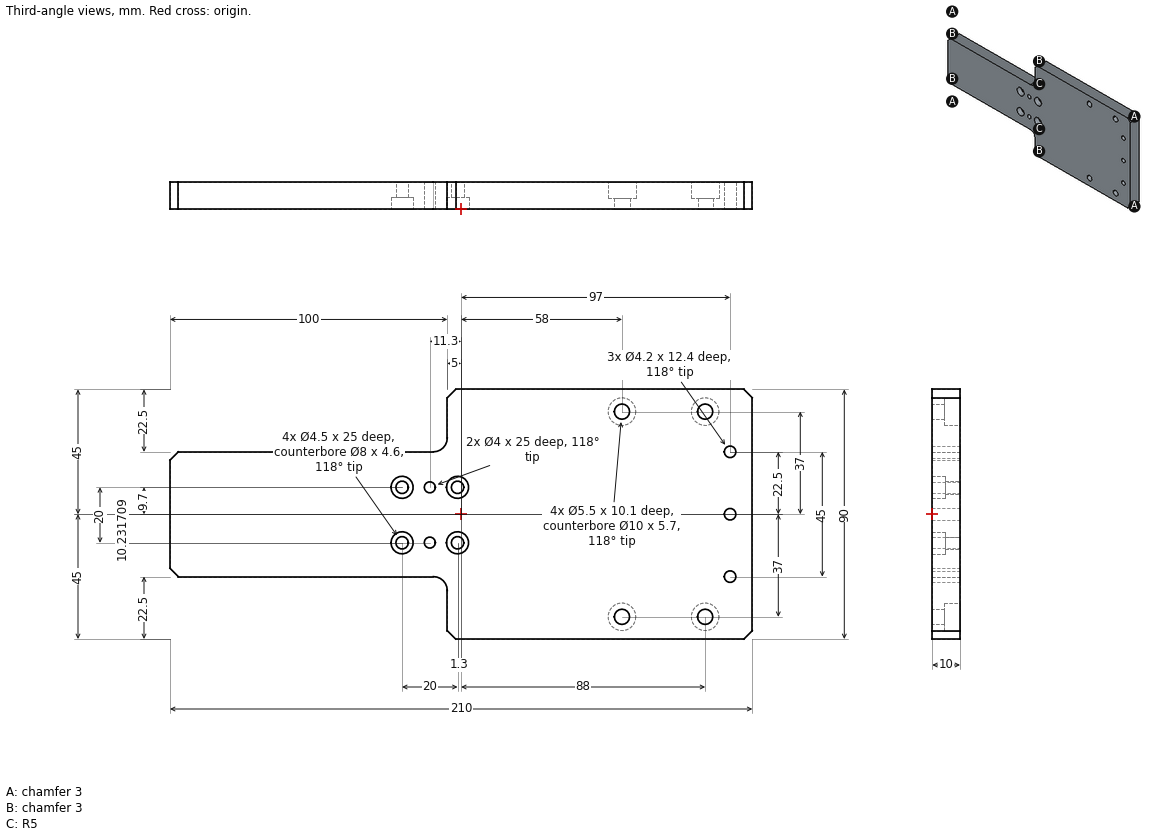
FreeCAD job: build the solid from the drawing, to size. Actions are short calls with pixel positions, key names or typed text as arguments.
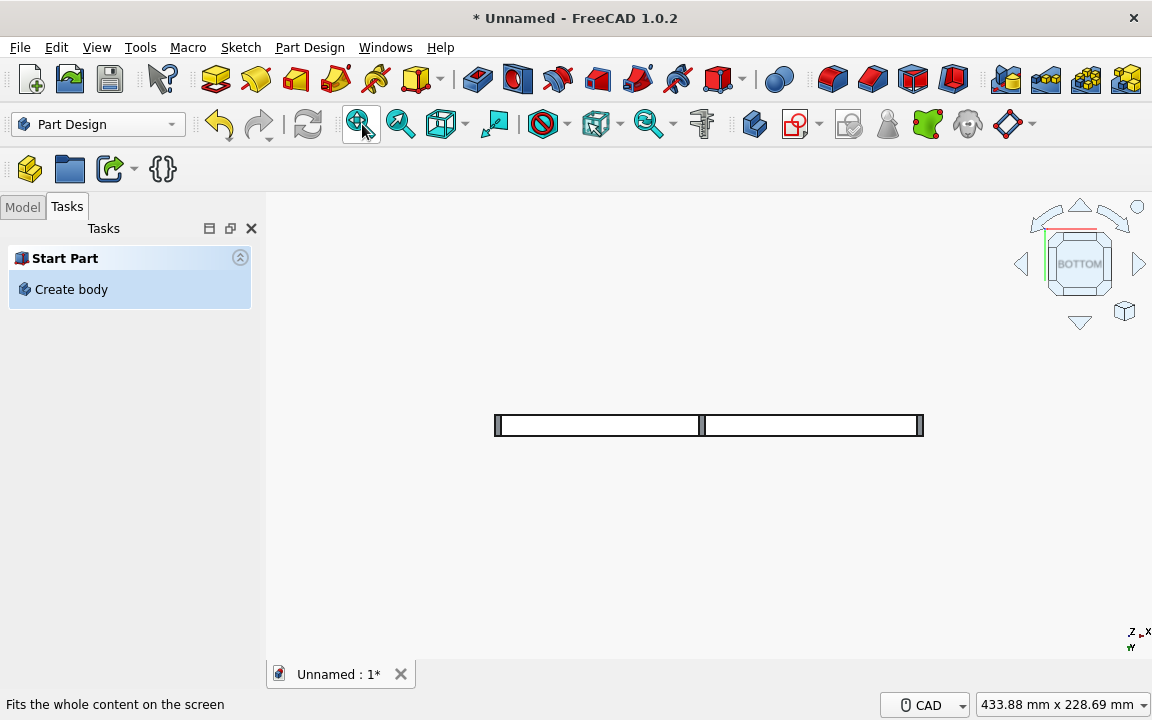
key(4)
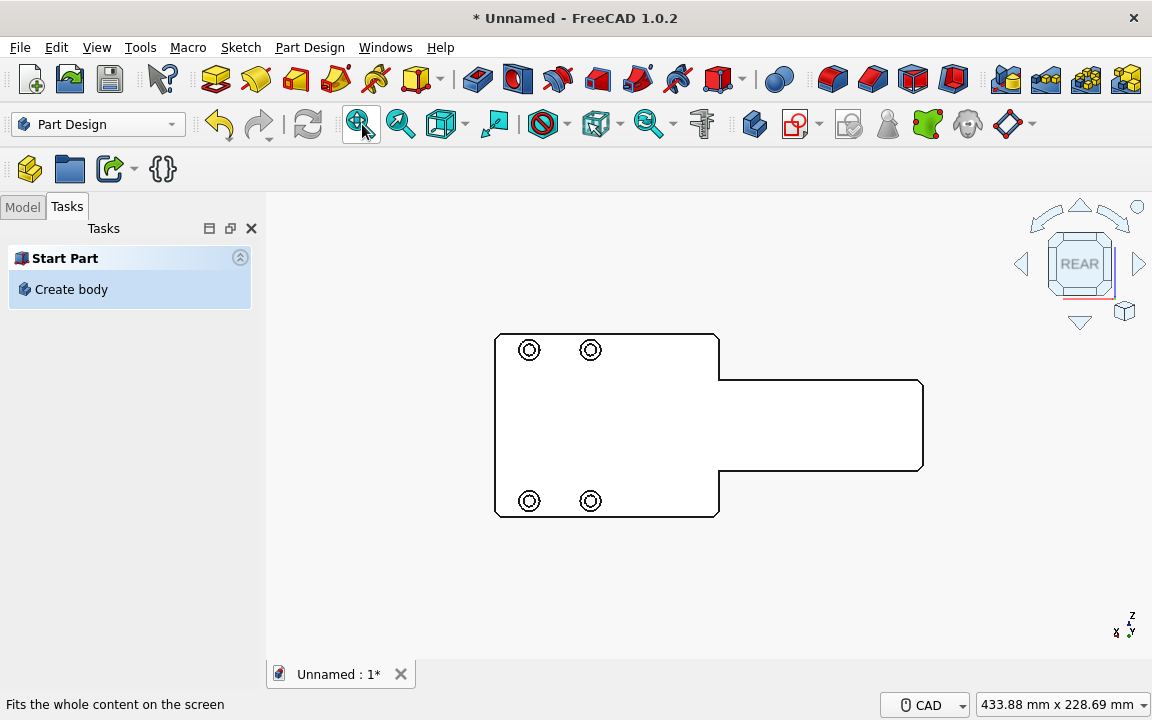
scroll(719, 379, up, 4)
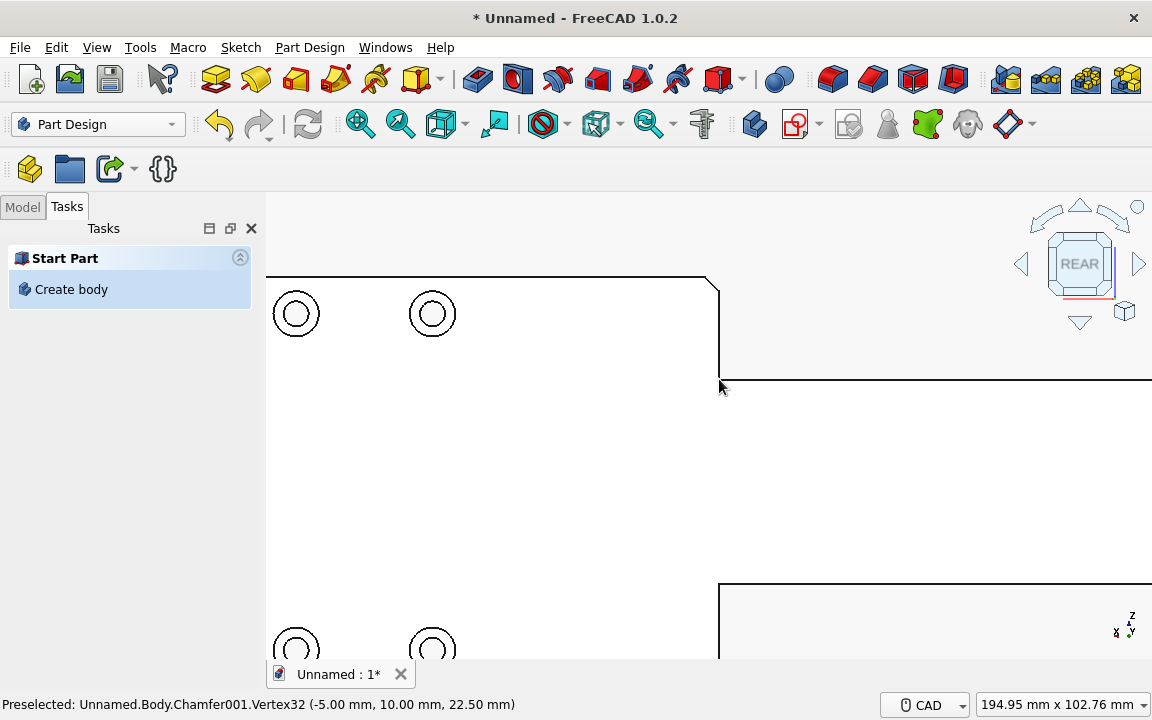
click(362, 124)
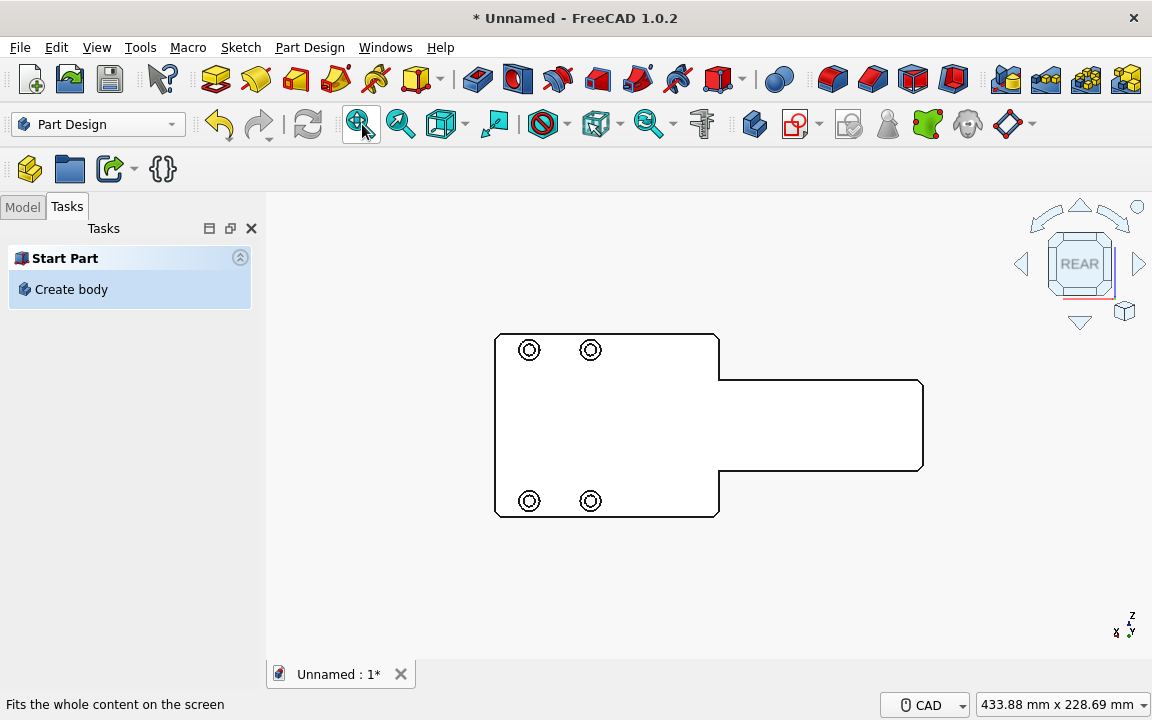
key(6)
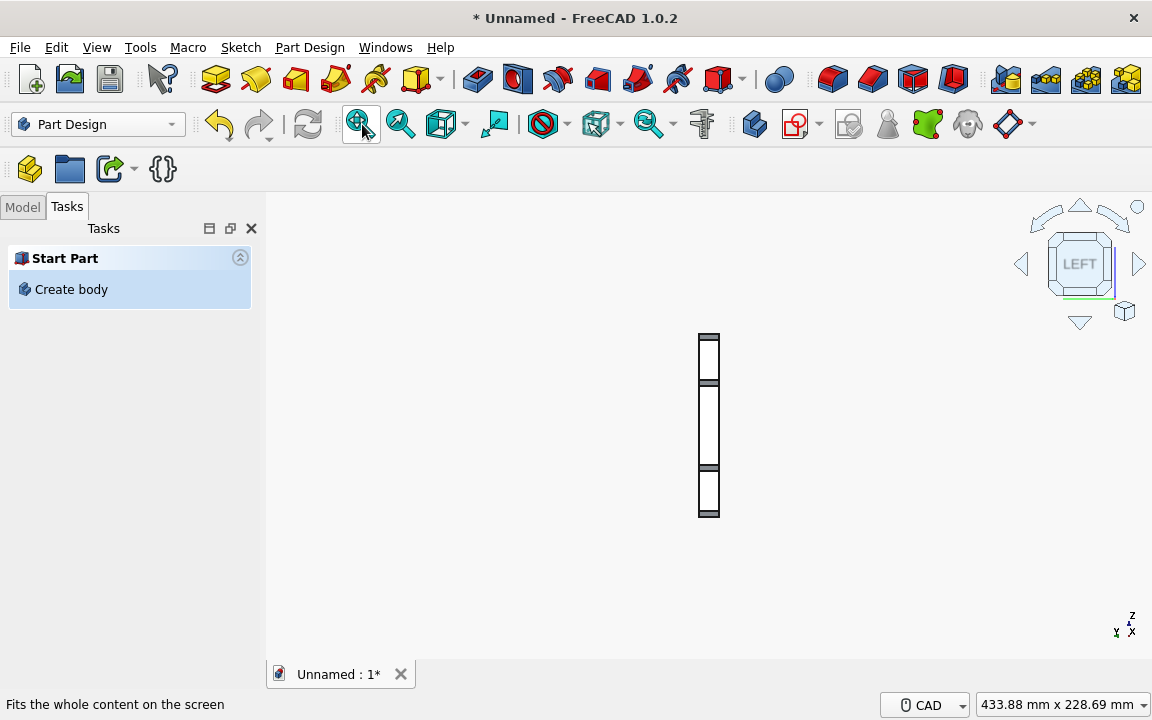
click(362, 124)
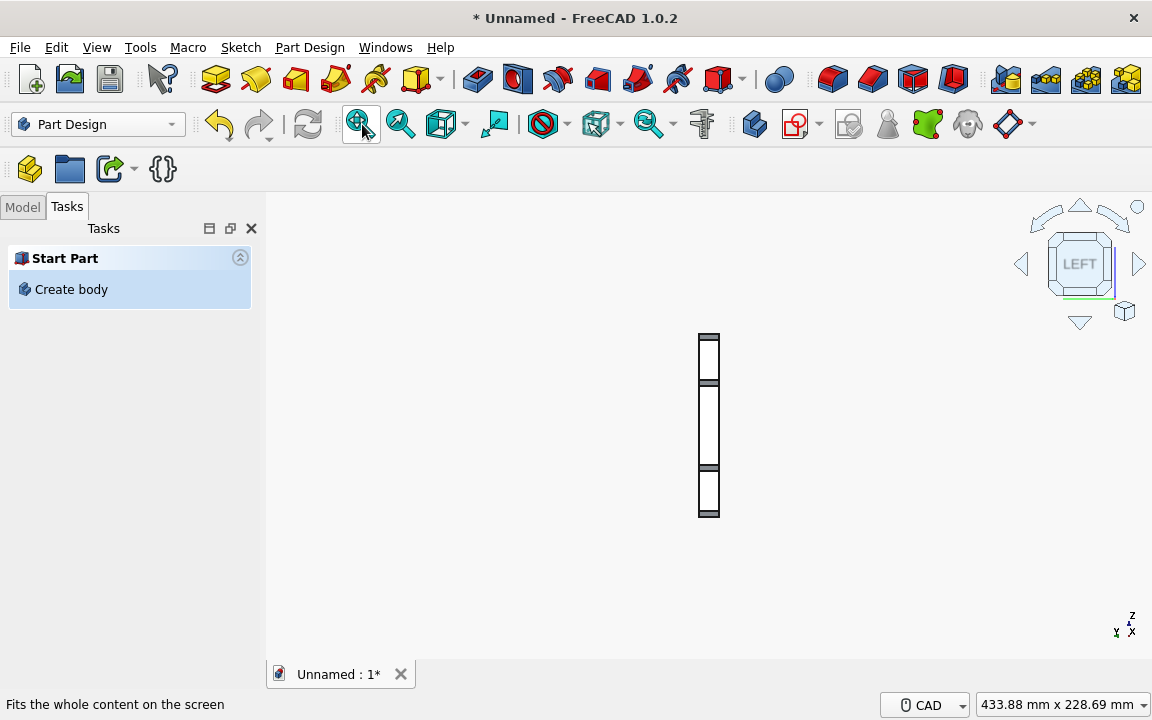
scroll(709, 379, up, 4)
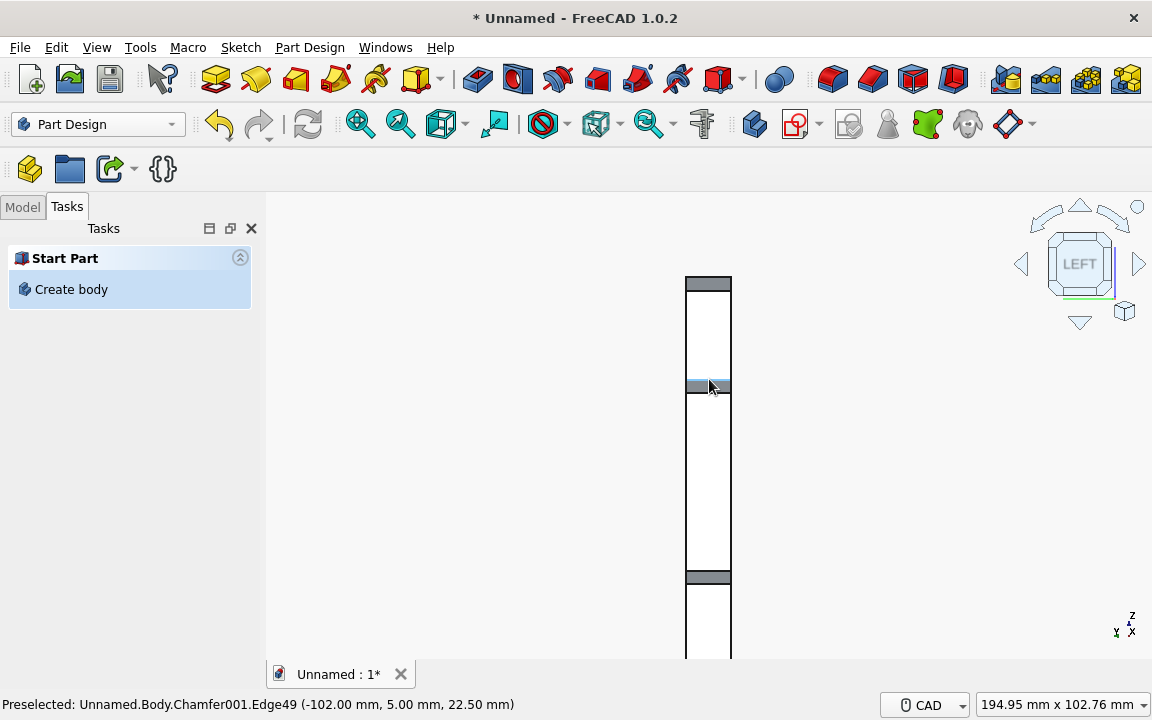
click(362, 124)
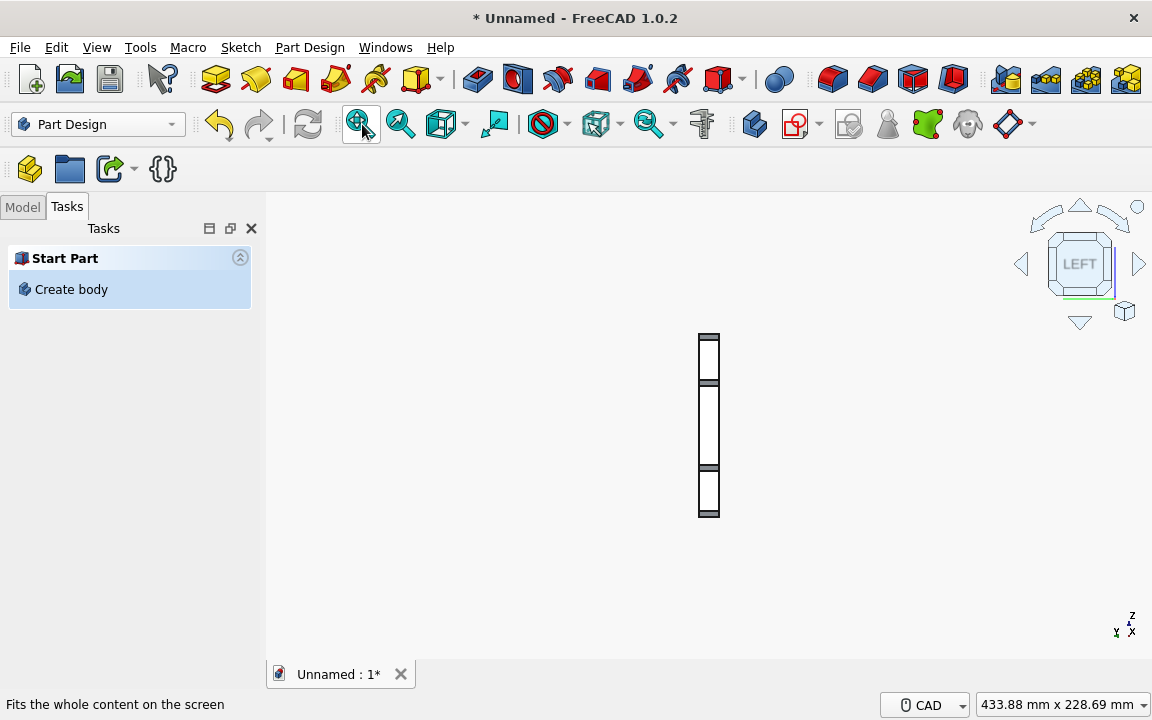
key(v)
key(3)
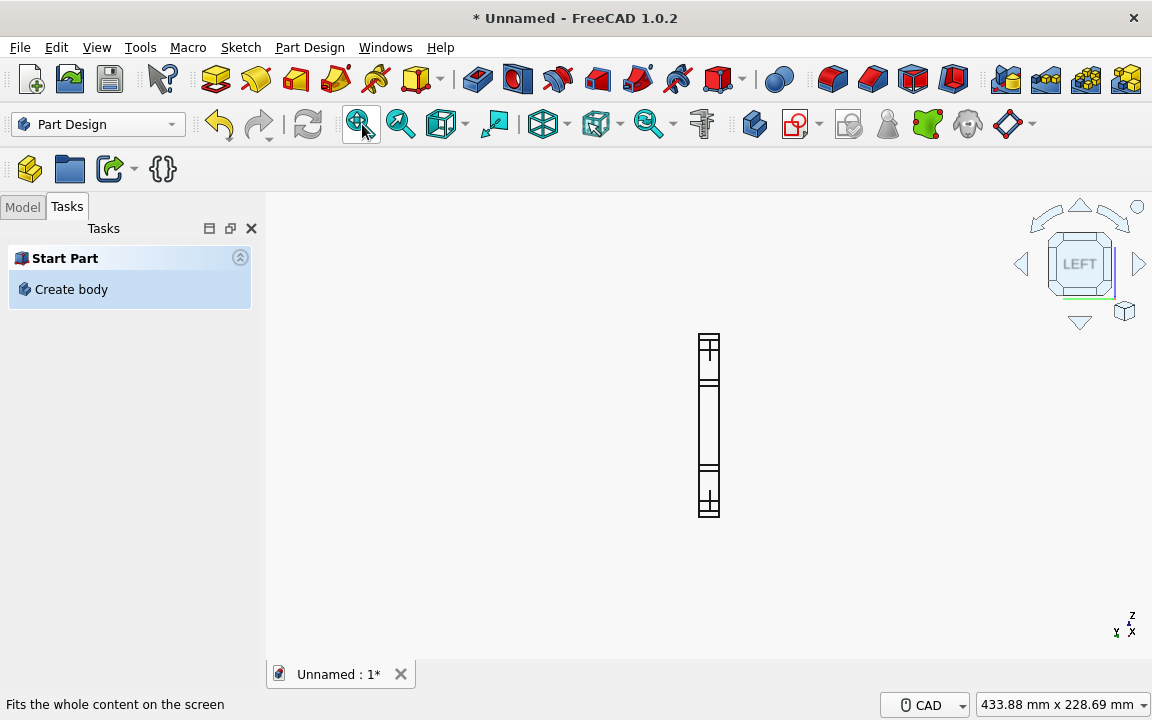
key(0)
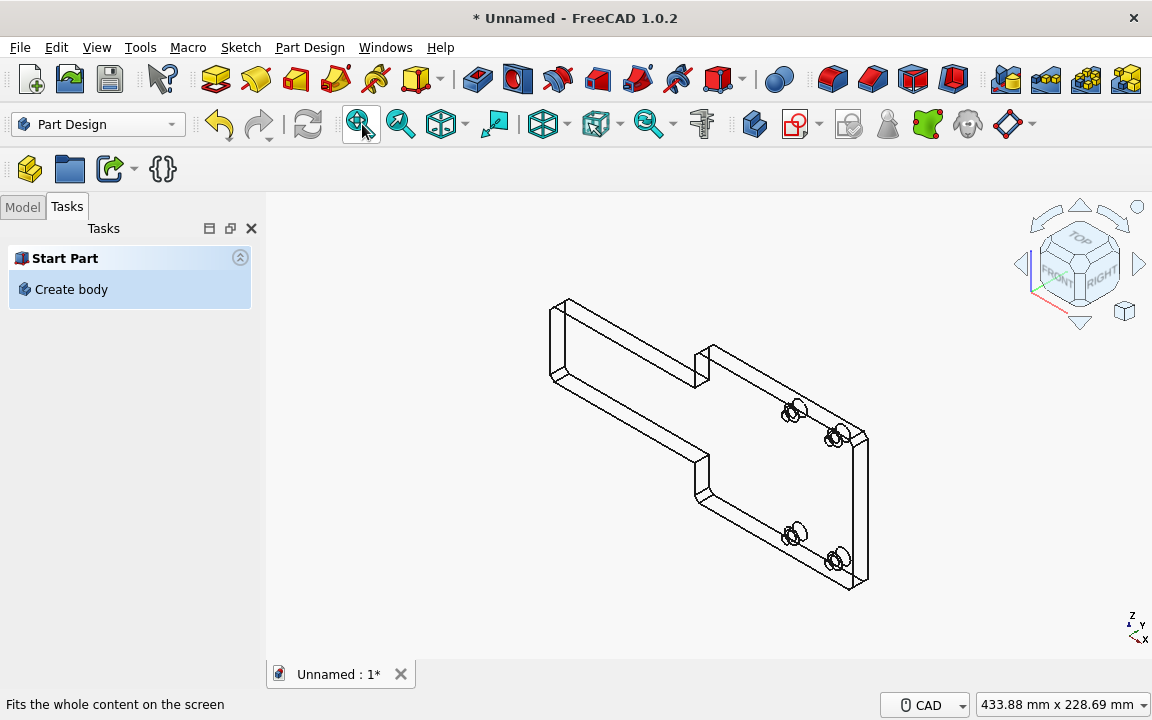
click(702, 383)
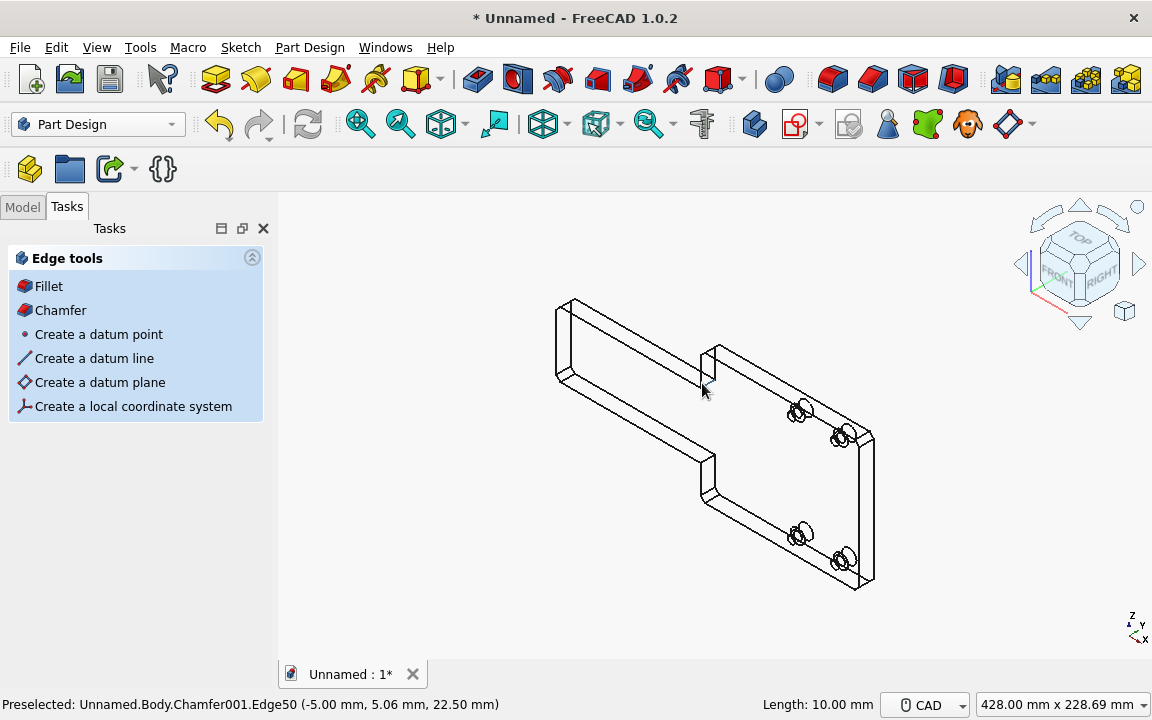
click(708, 458, ctrl)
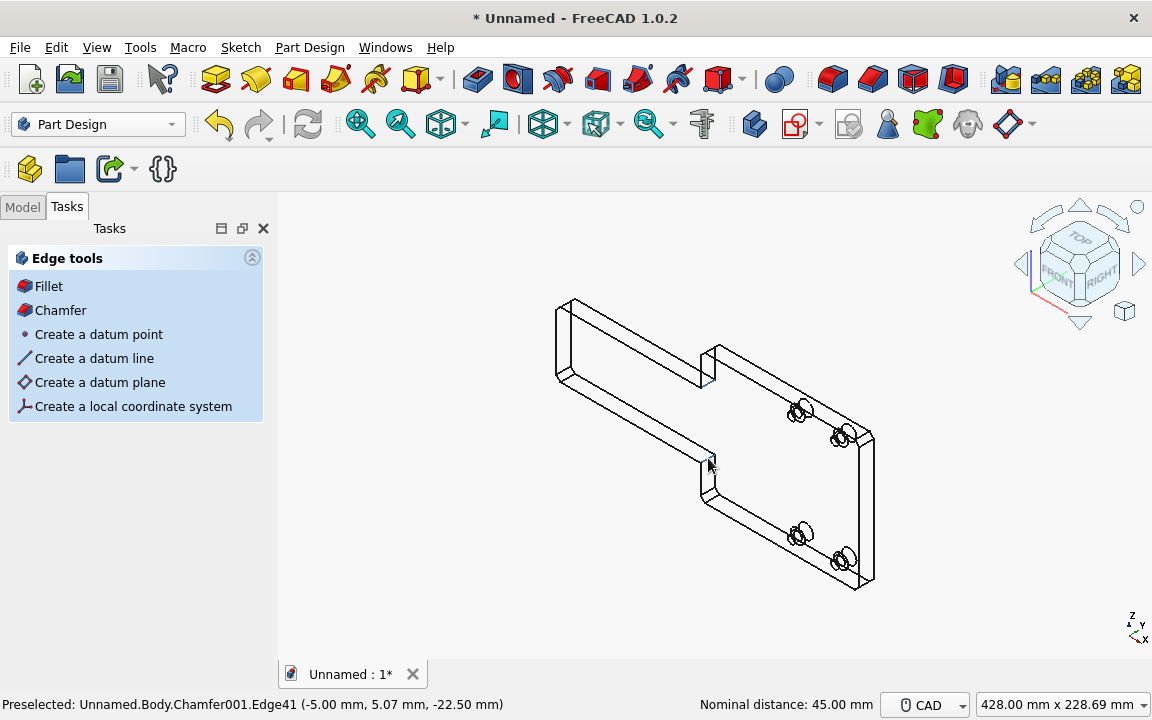
key(v)
key(1)